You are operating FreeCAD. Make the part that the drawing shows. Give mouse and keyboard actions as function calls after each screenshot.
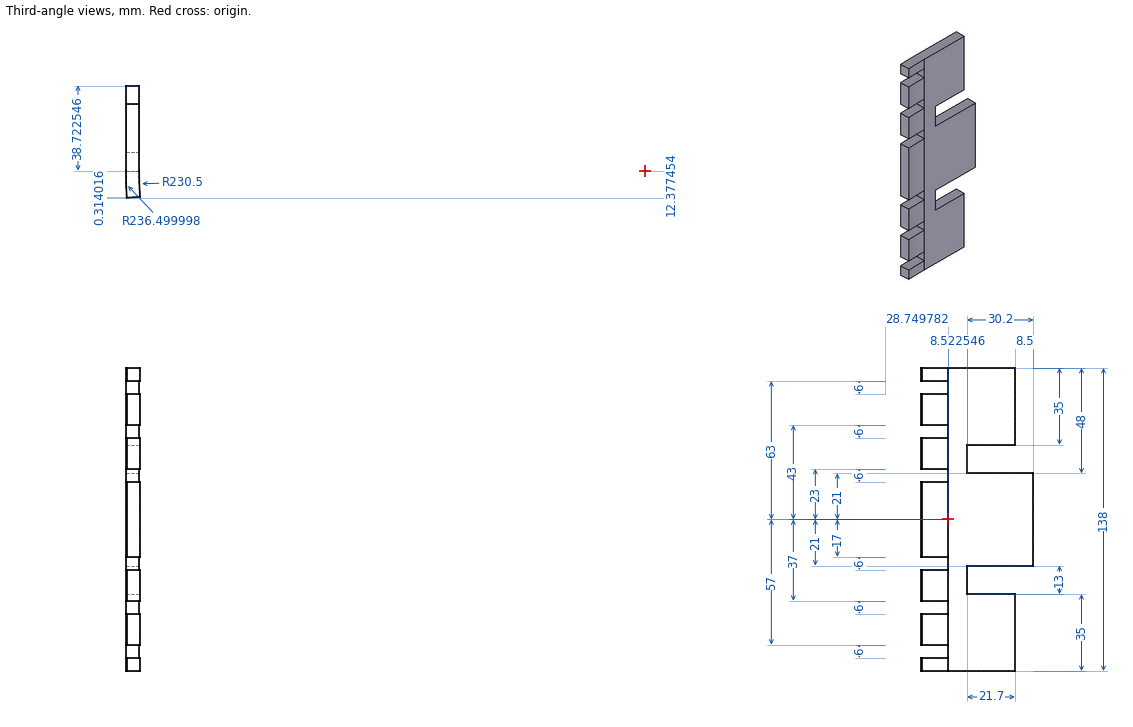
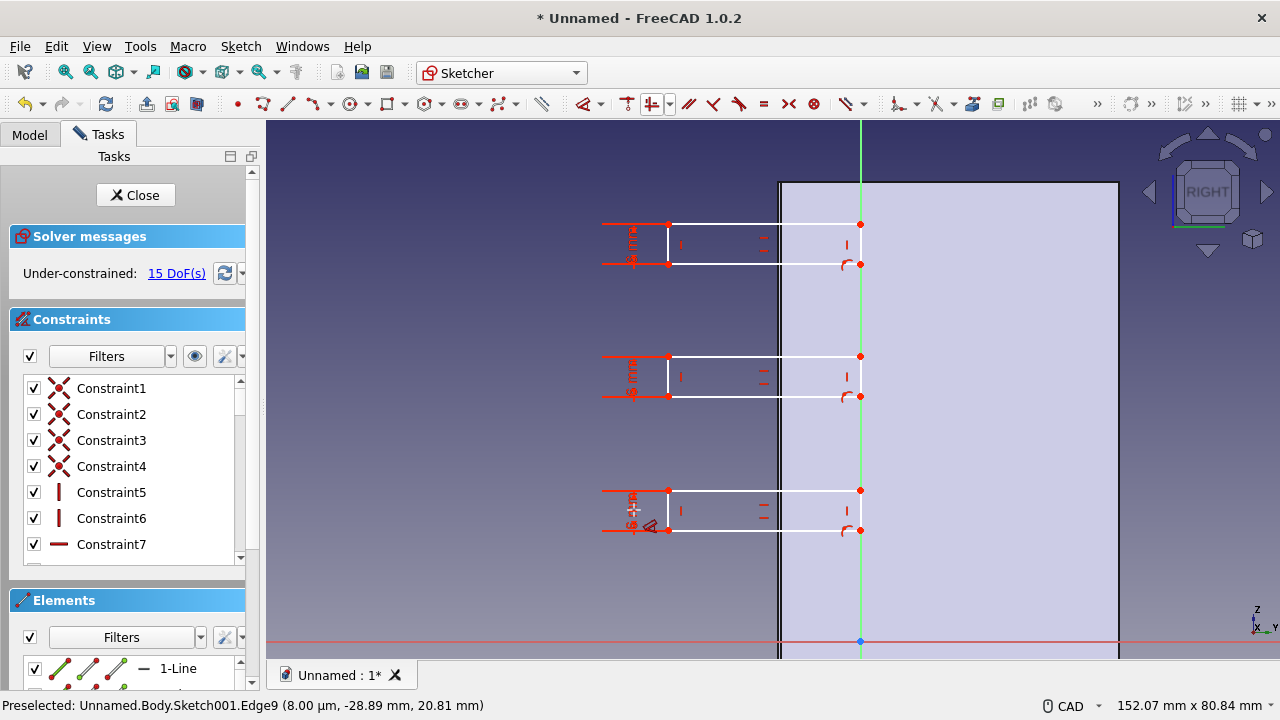
scroll(669, 243, down, 5)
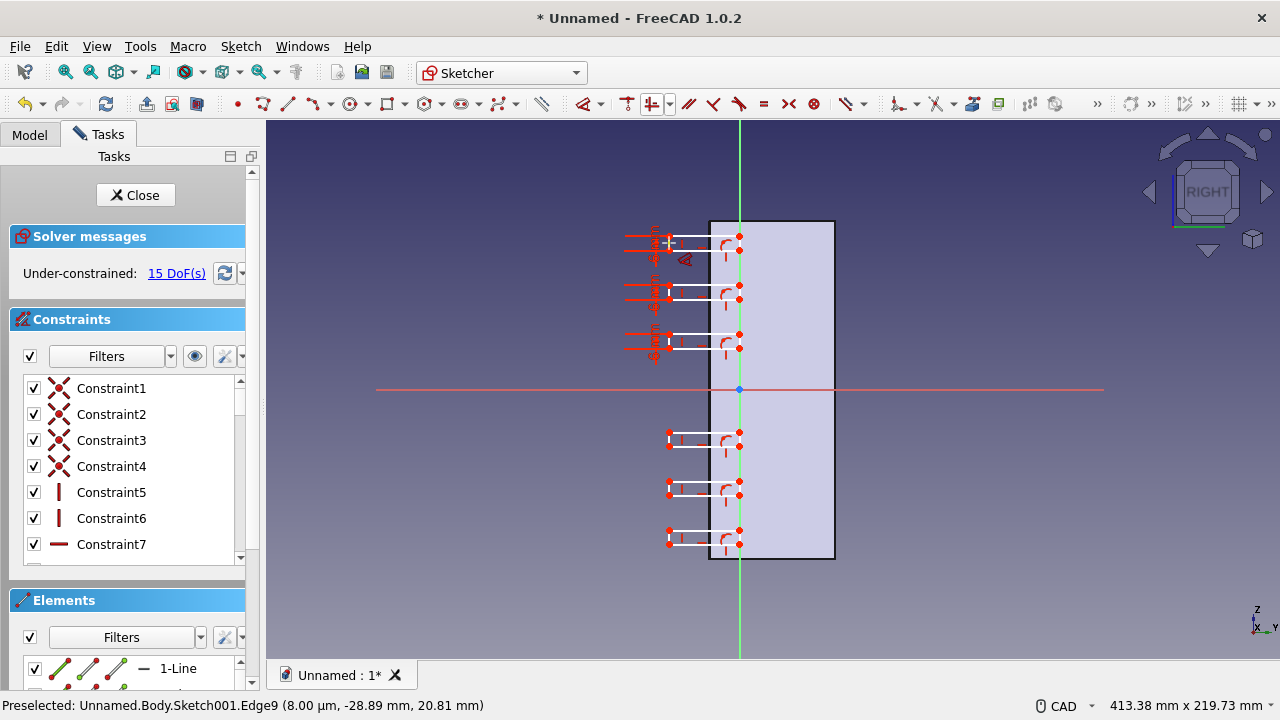
scroll(669, 437, up, 6)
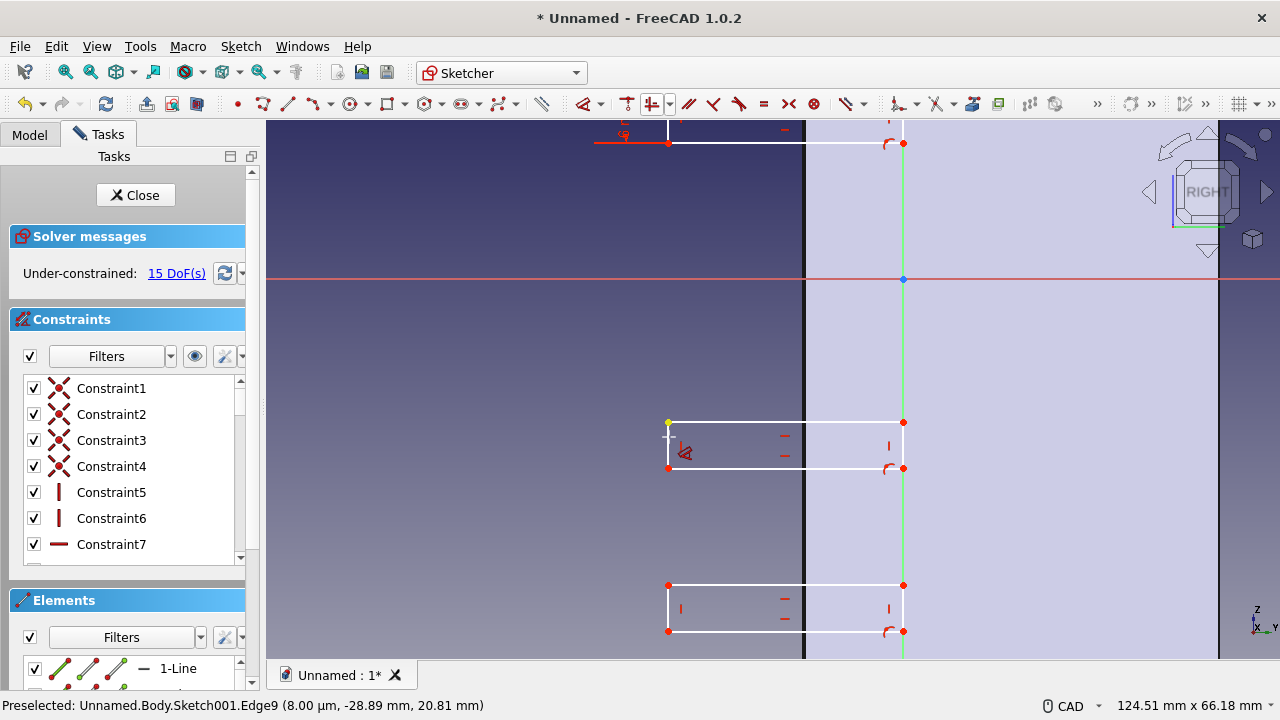
click(668, 436)
click(634, 446)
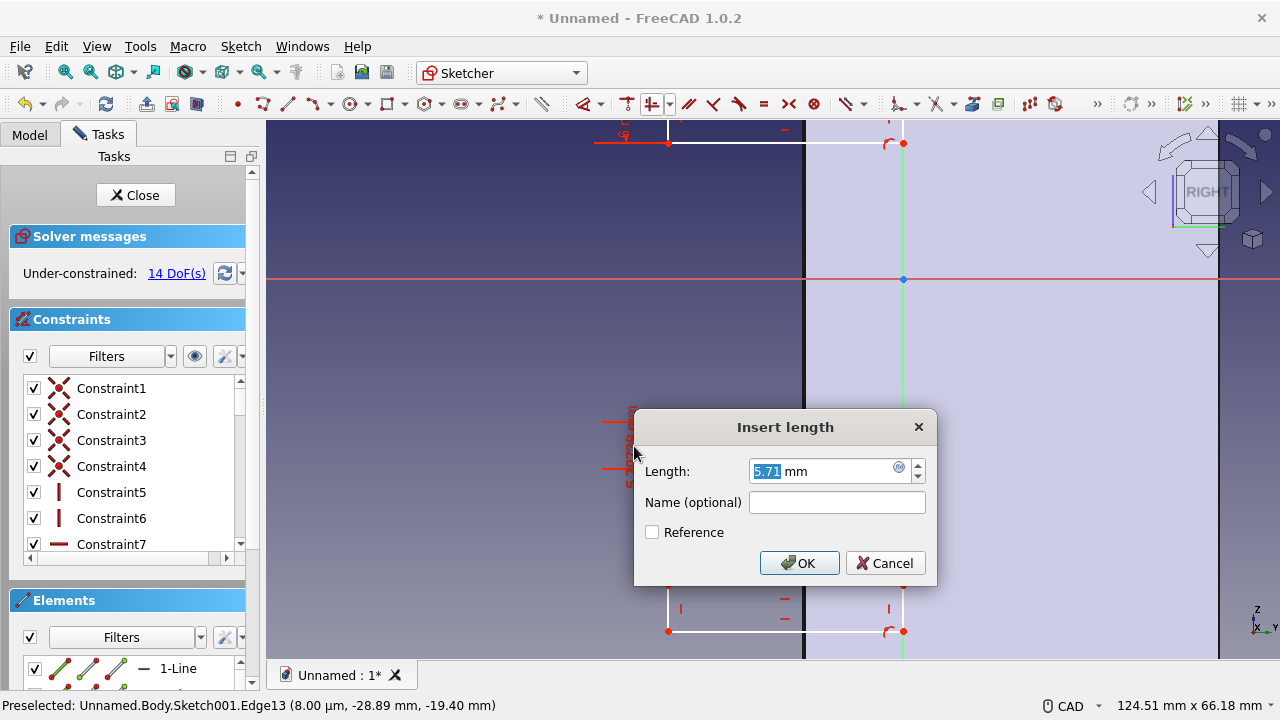
text(6)
key(Return)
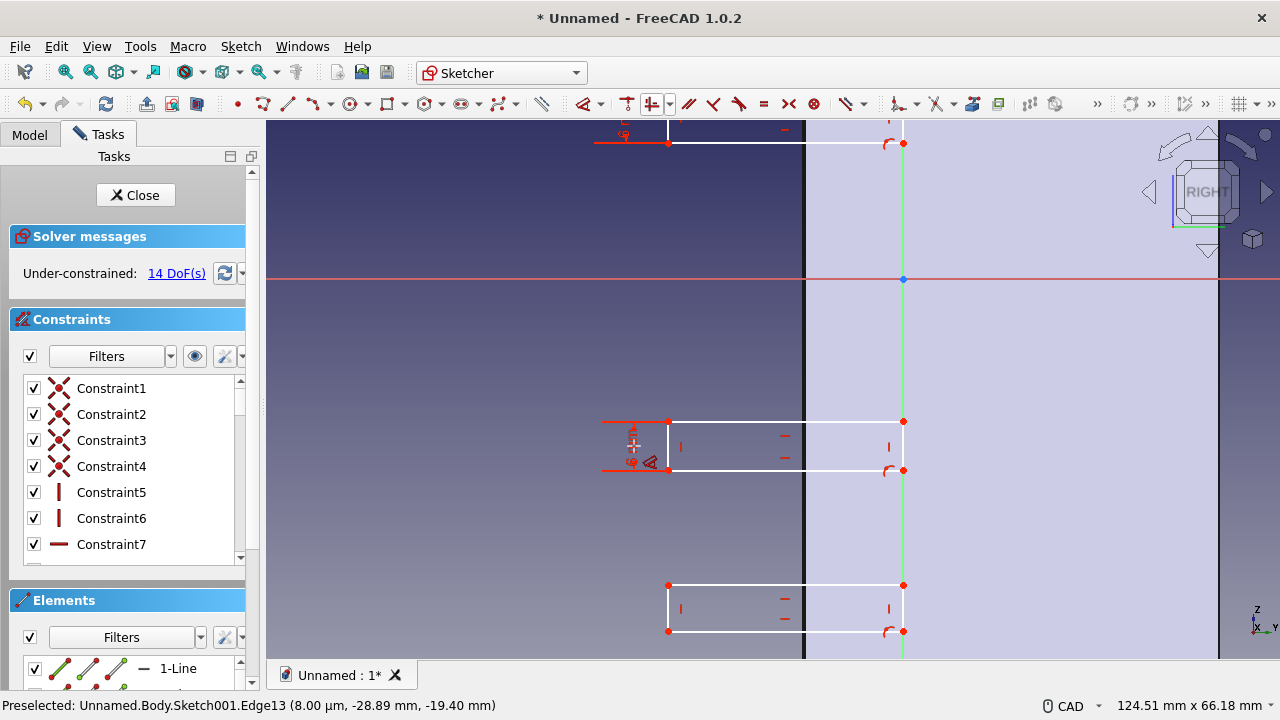
click(668, 599)
click(634, 608)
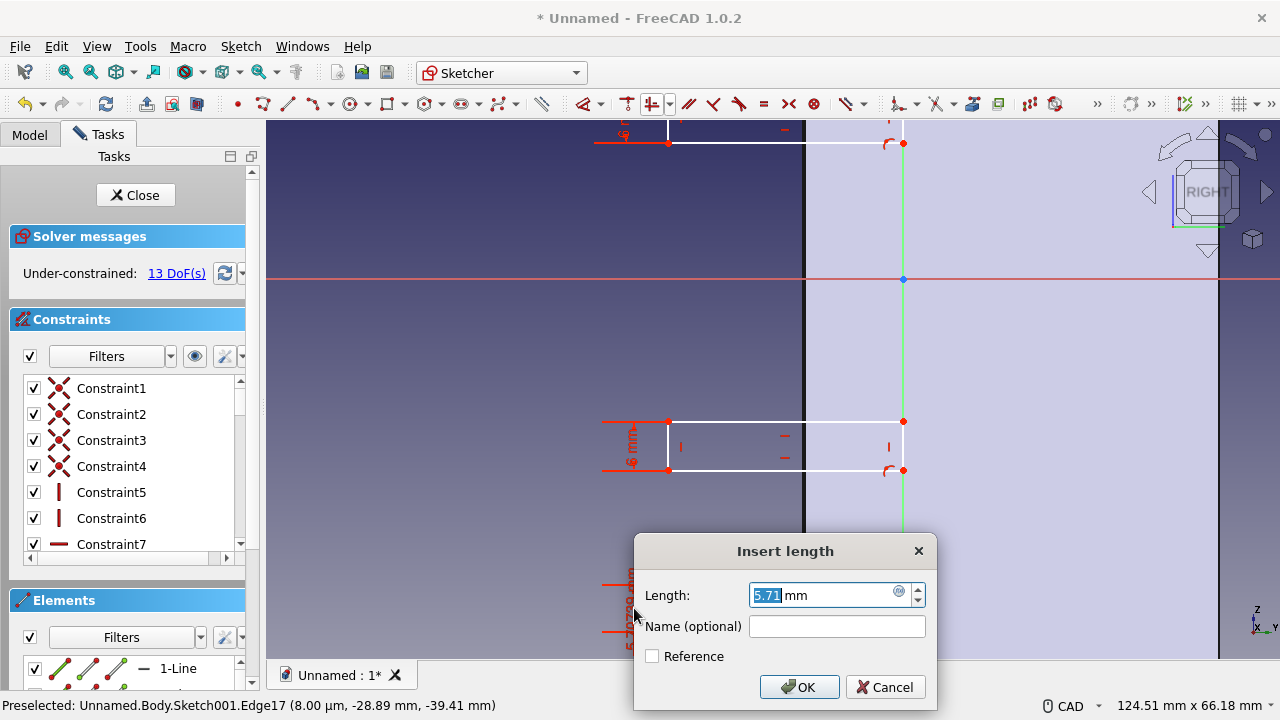
text(6)
key(Return)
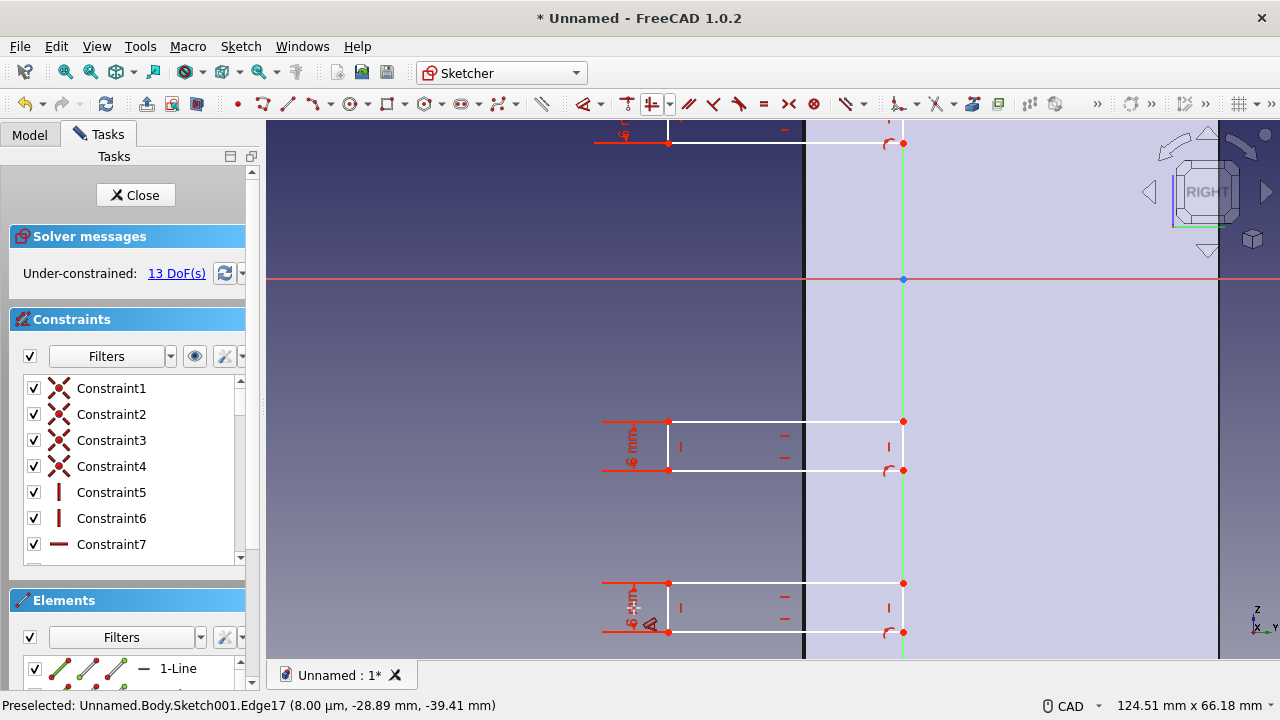
scroll(669, 437, down, 6)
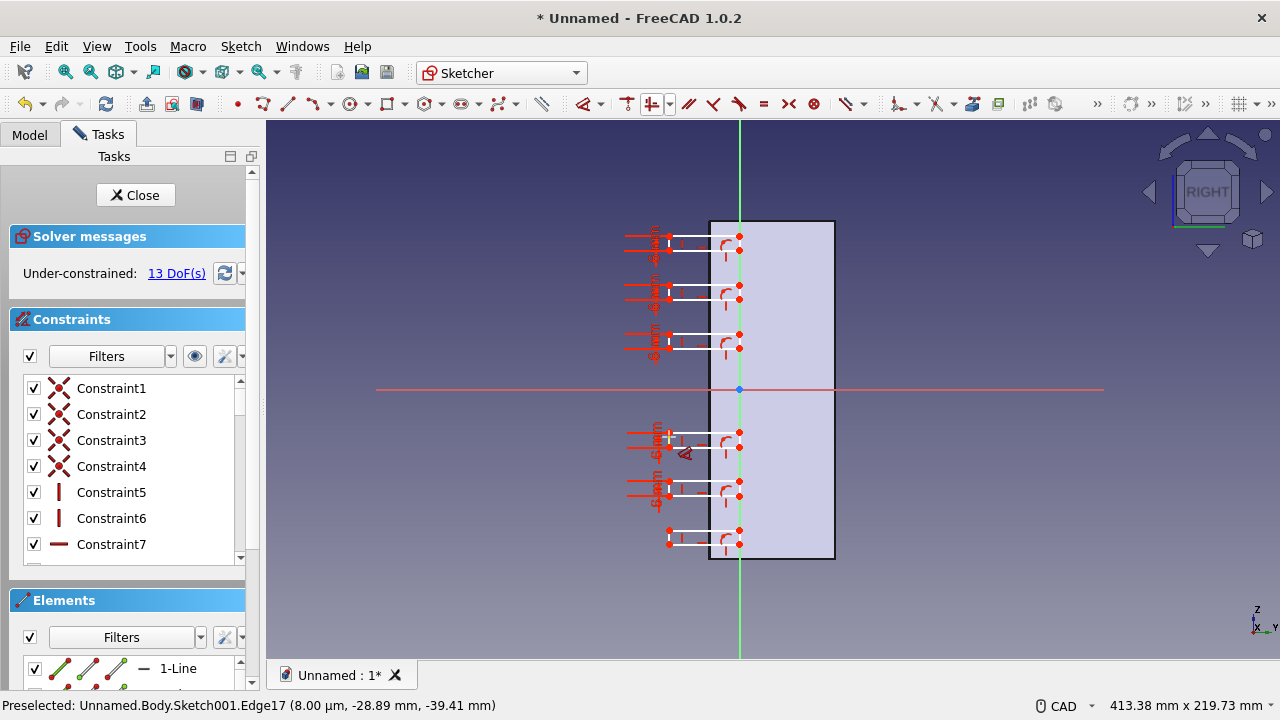
scroll(669, 535, up, 6)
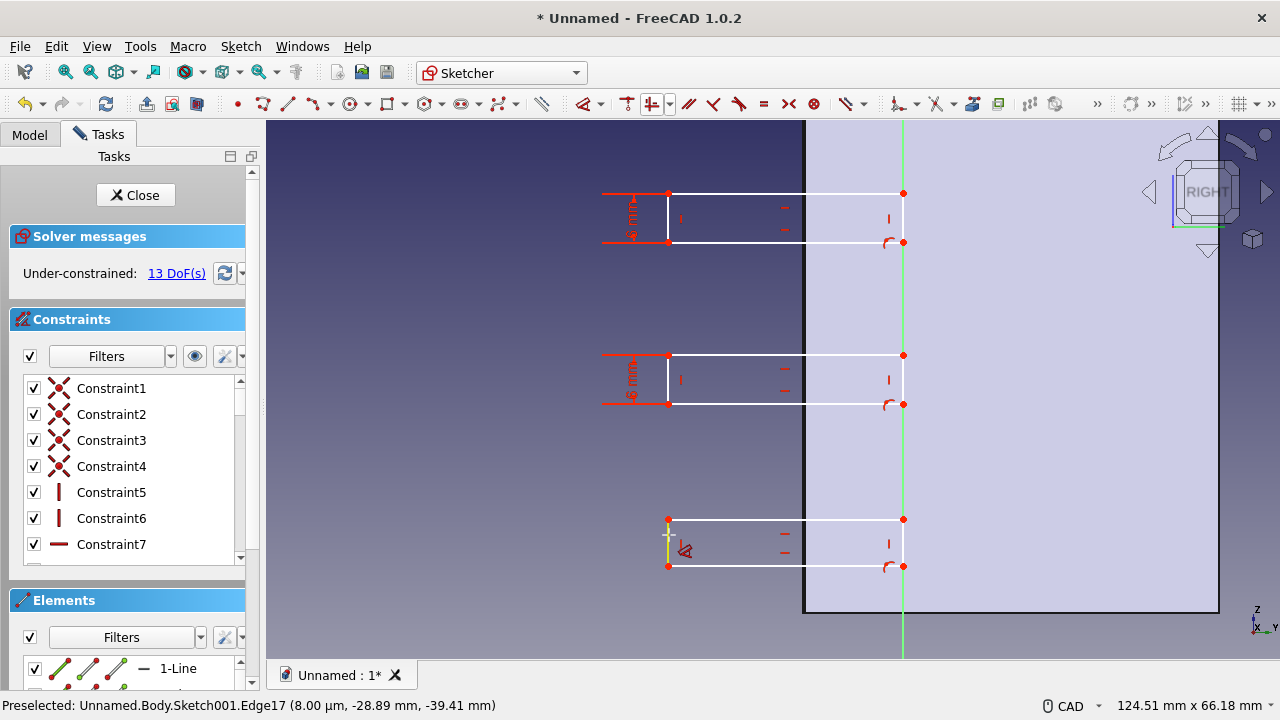
click(668, 534)
click(634, 543)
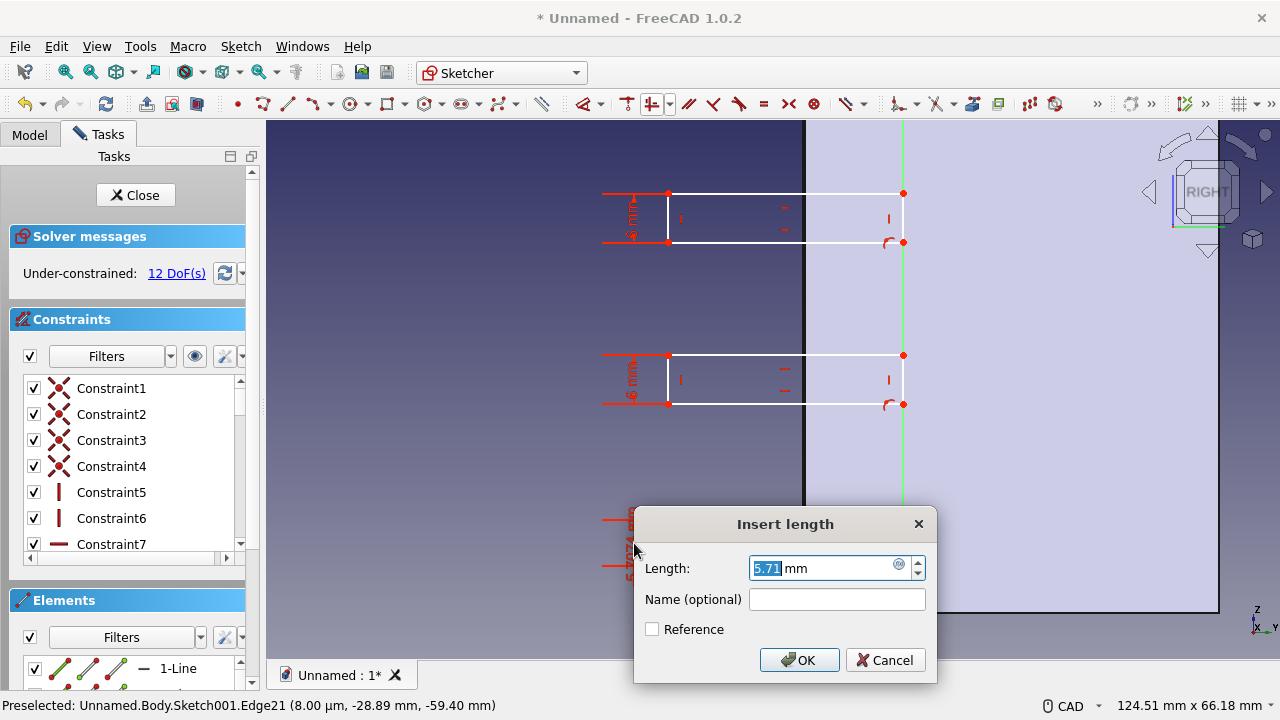
text(6)
key(Return)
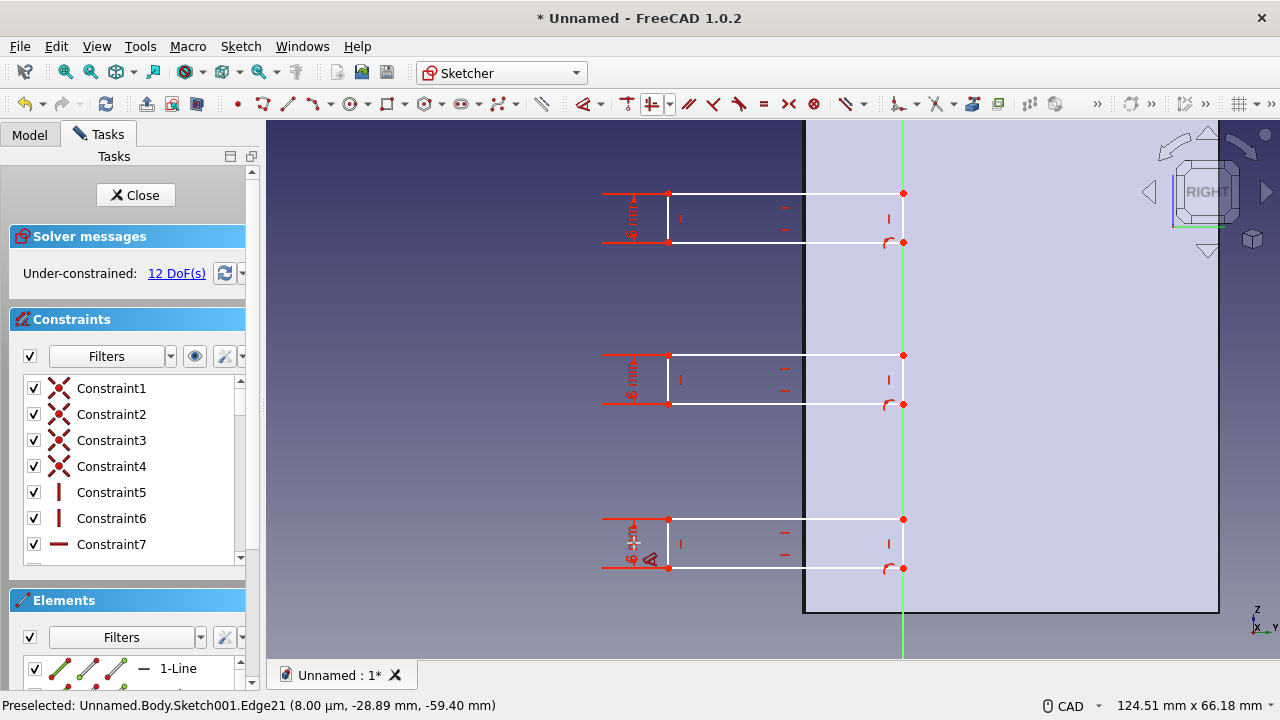
scroll(669, 535, down, 6)